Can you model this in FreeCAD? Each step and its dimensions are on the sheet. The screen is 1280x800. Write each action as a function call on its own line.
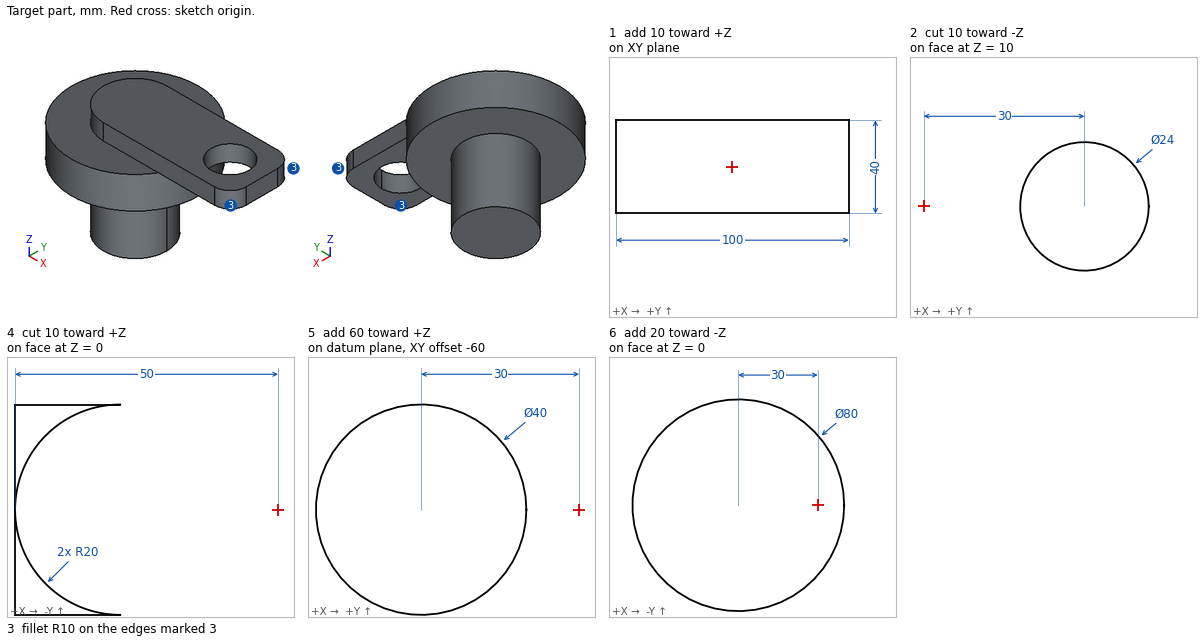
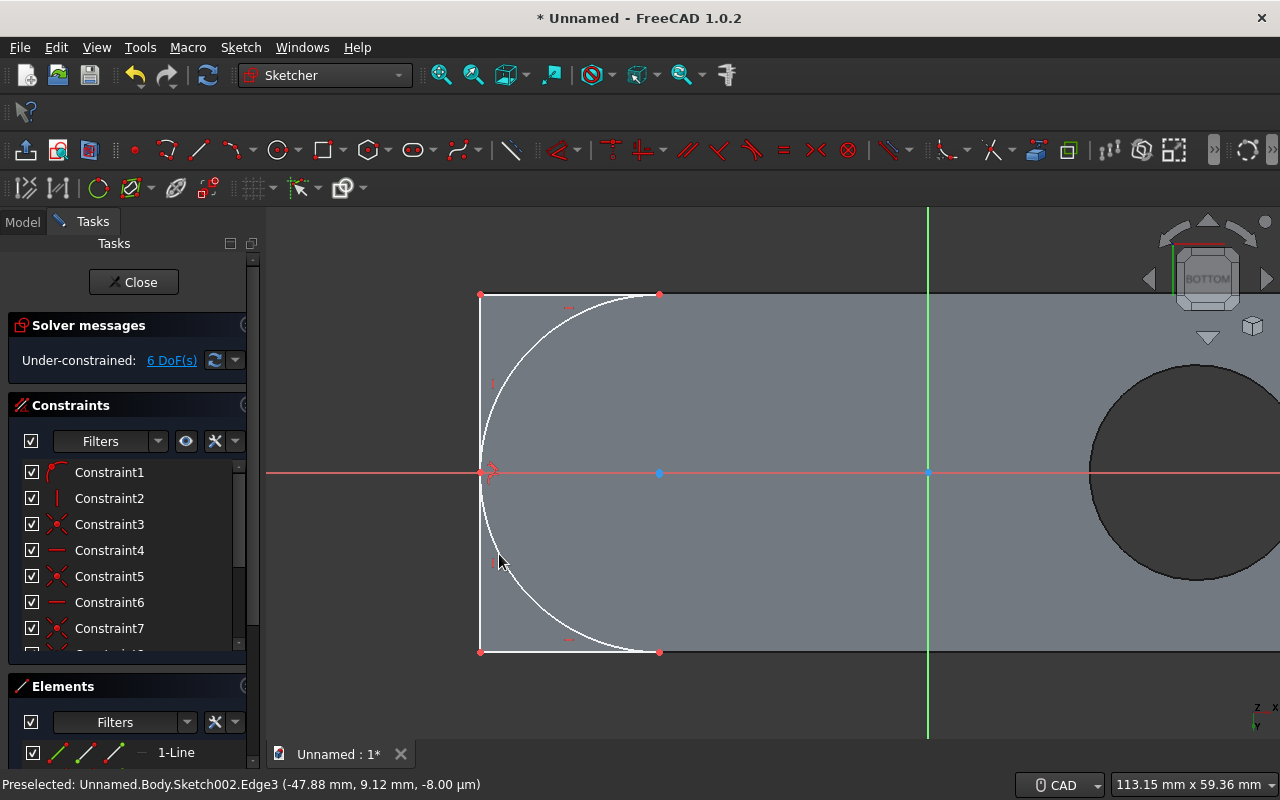
click(480, 598)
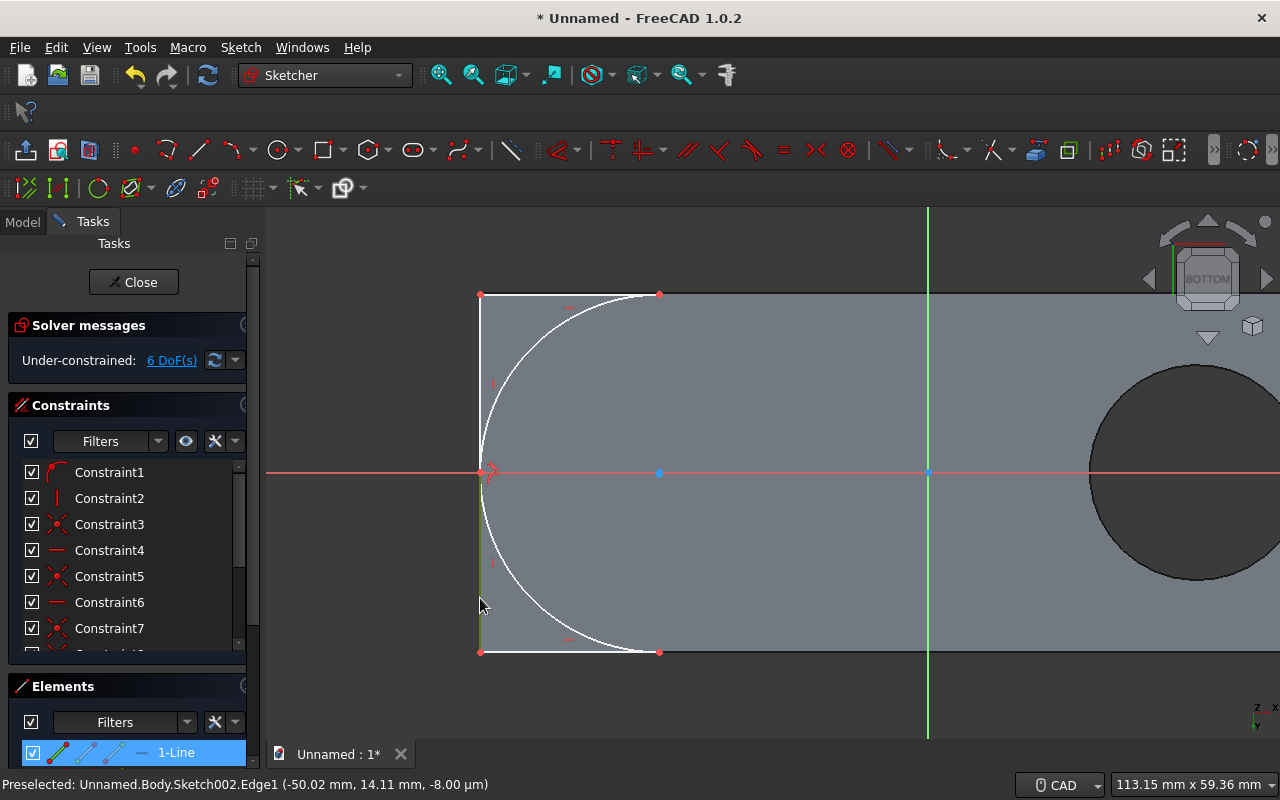
click(578, 314)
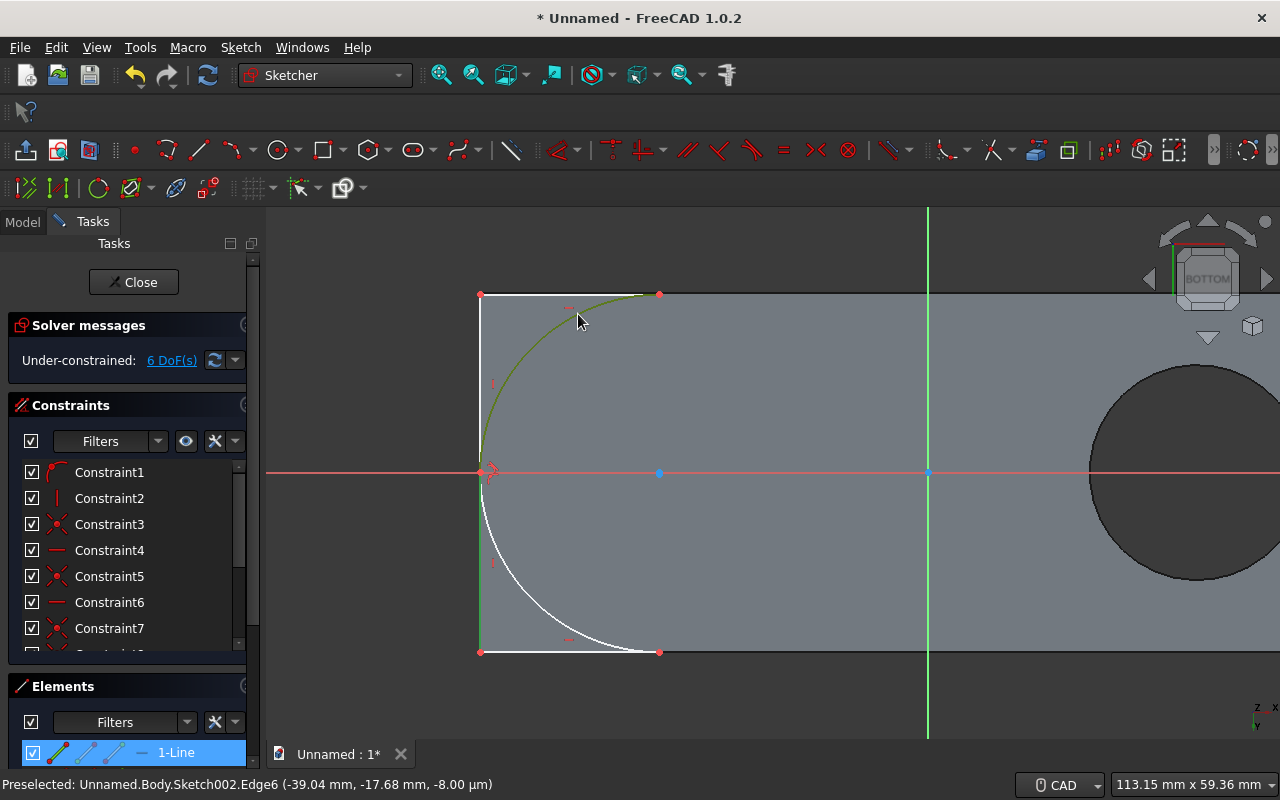
click(752, 150)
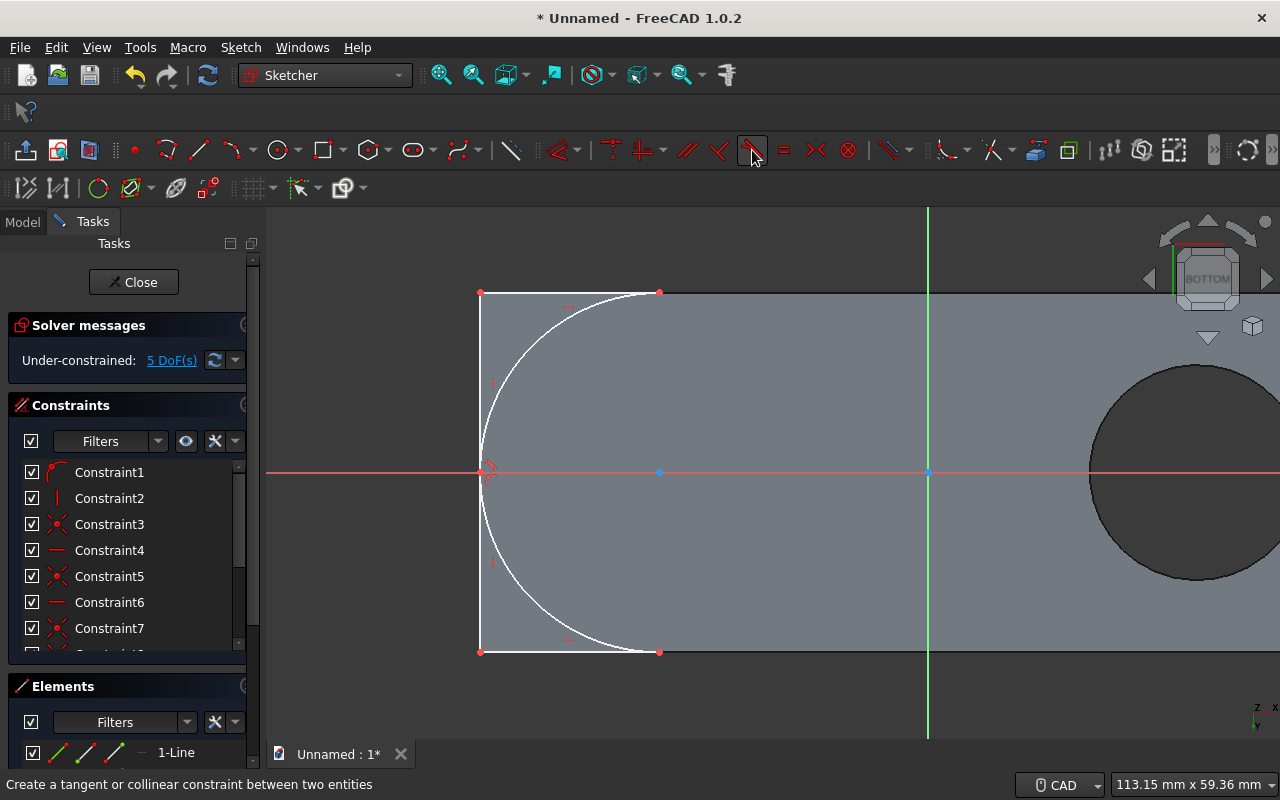
click(534, 652)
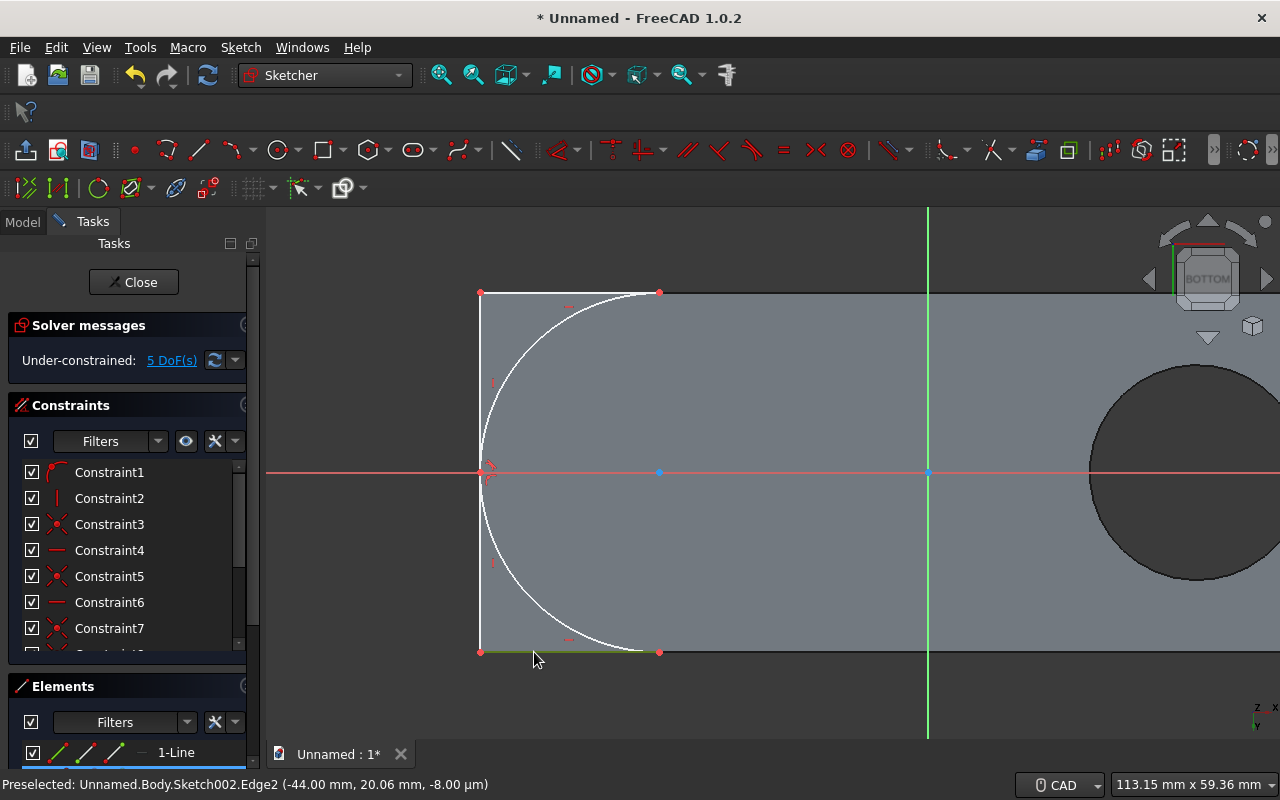
click(500, 554)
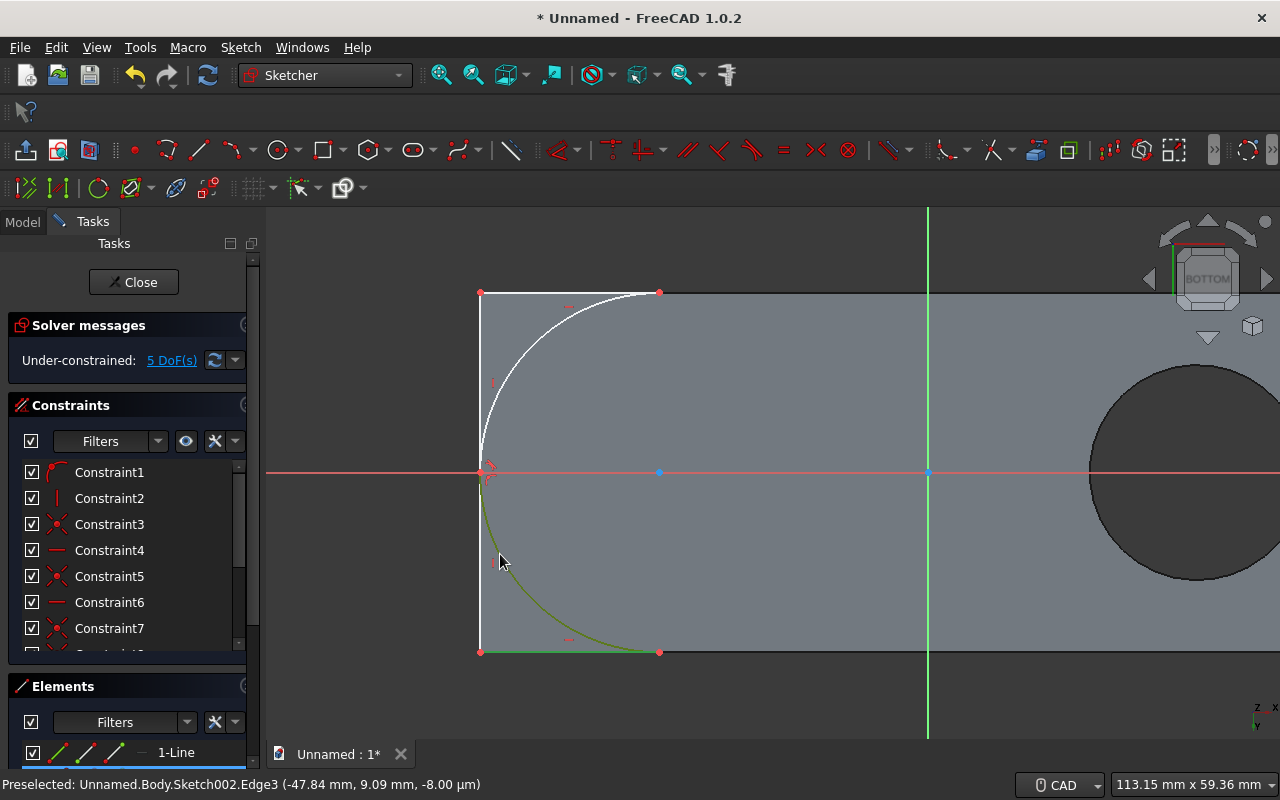
click(752, 150)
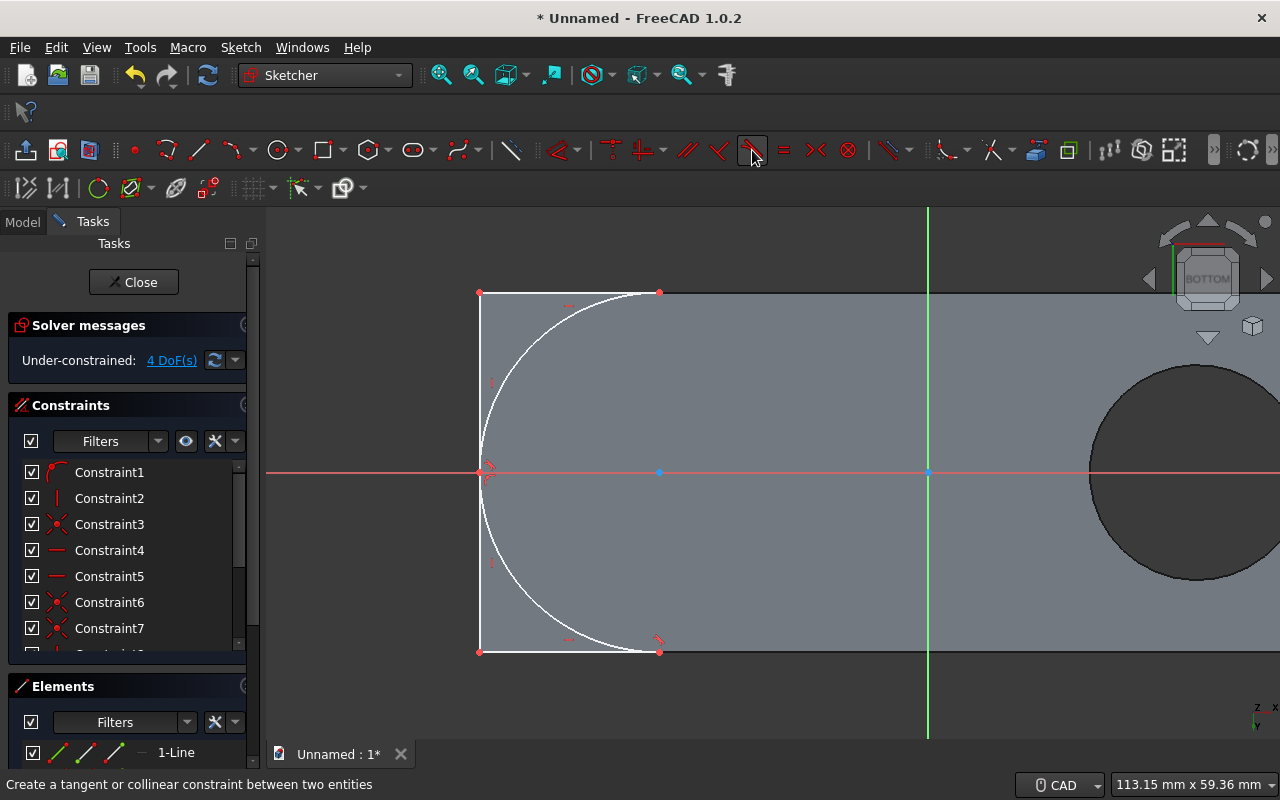
click(534, 293)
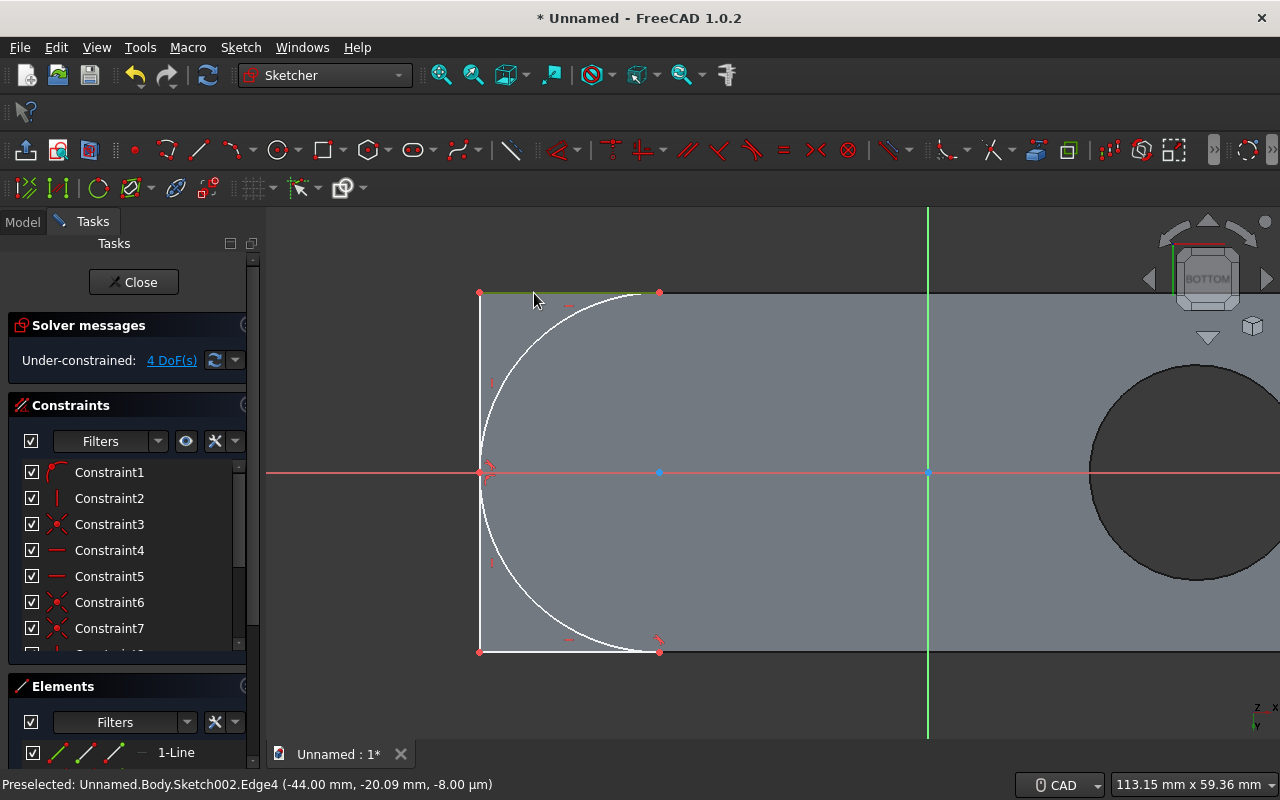
click(578, 312)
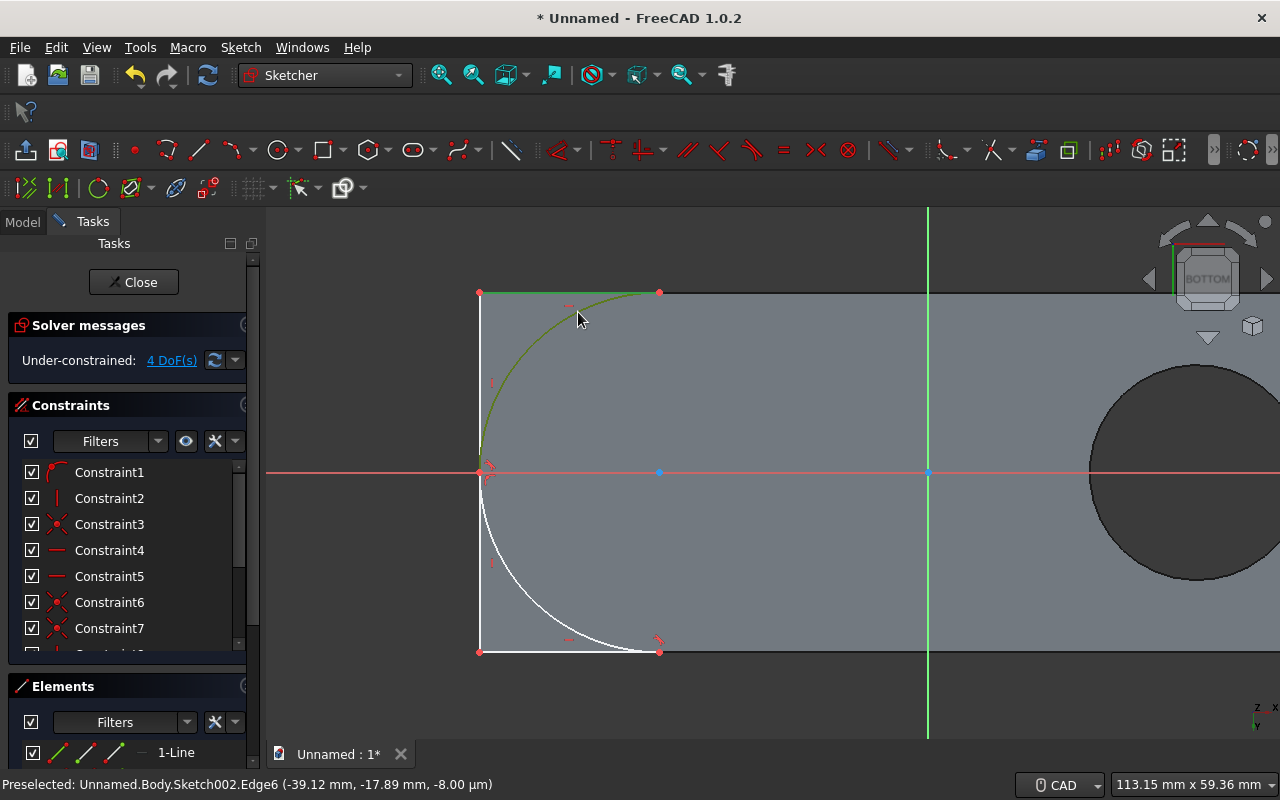
click(752, 150)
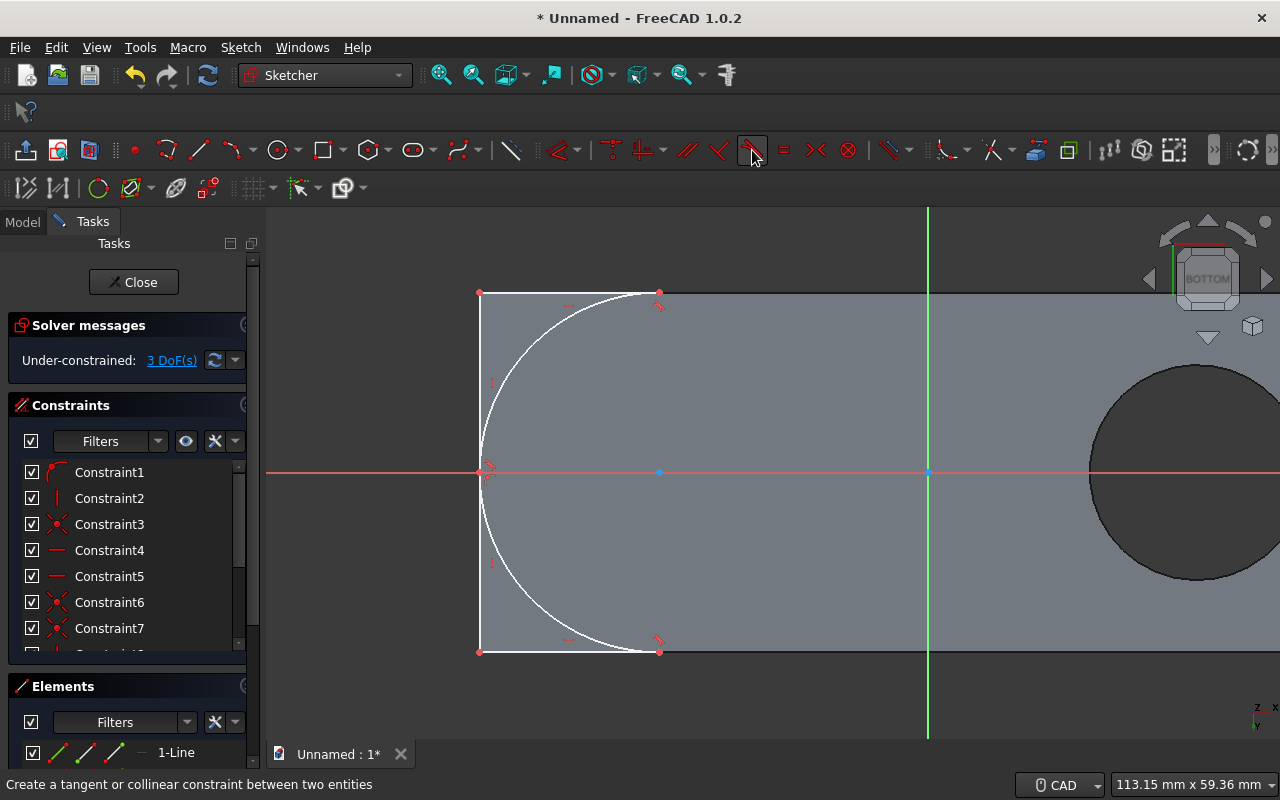
click(499, 554)